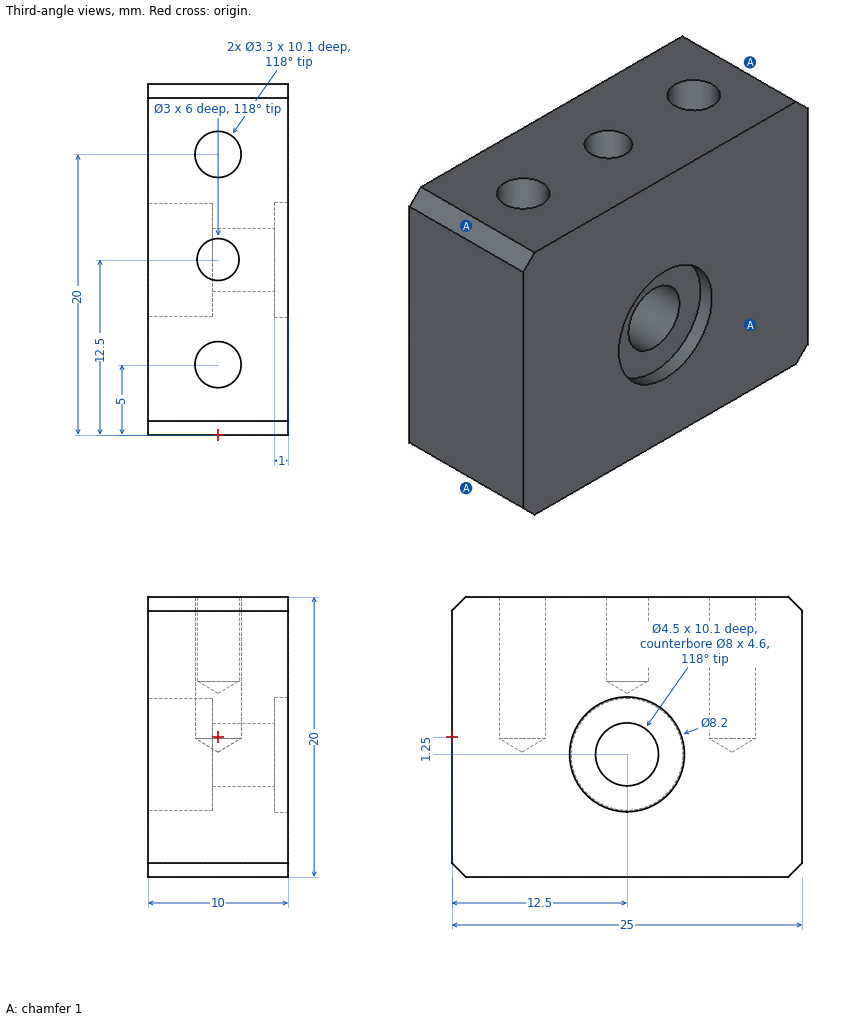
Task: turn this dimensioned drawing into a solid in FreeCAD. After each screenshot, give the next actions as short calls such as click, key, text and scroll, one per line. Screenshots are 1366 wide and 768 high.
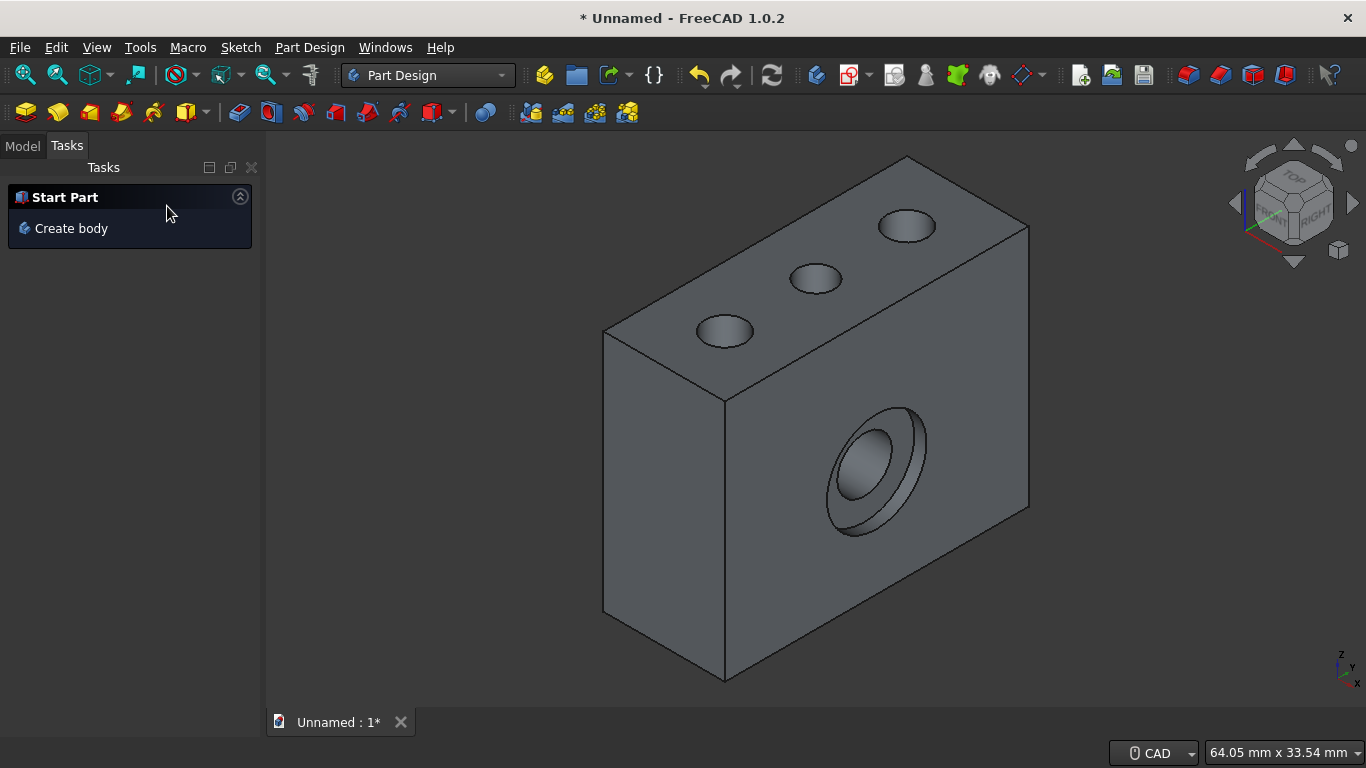
click(664, 365)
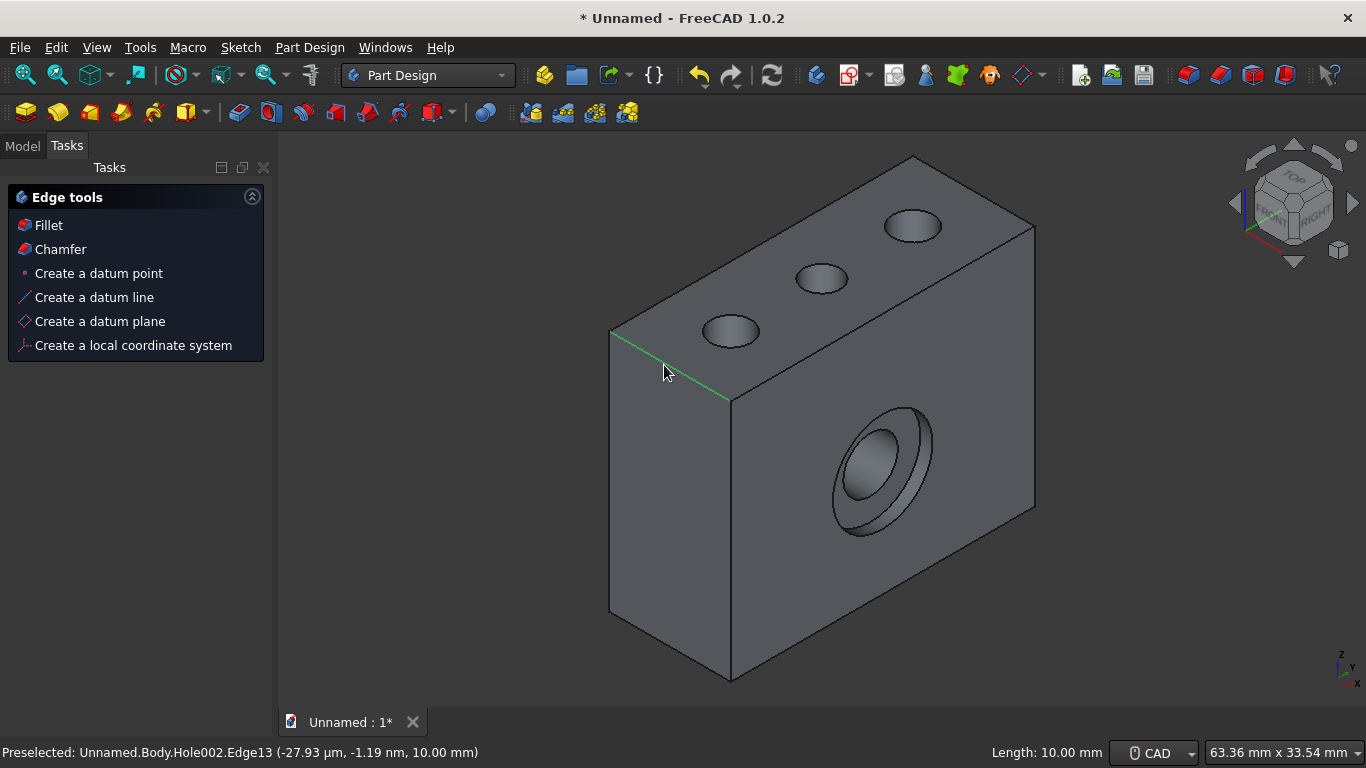
key(2)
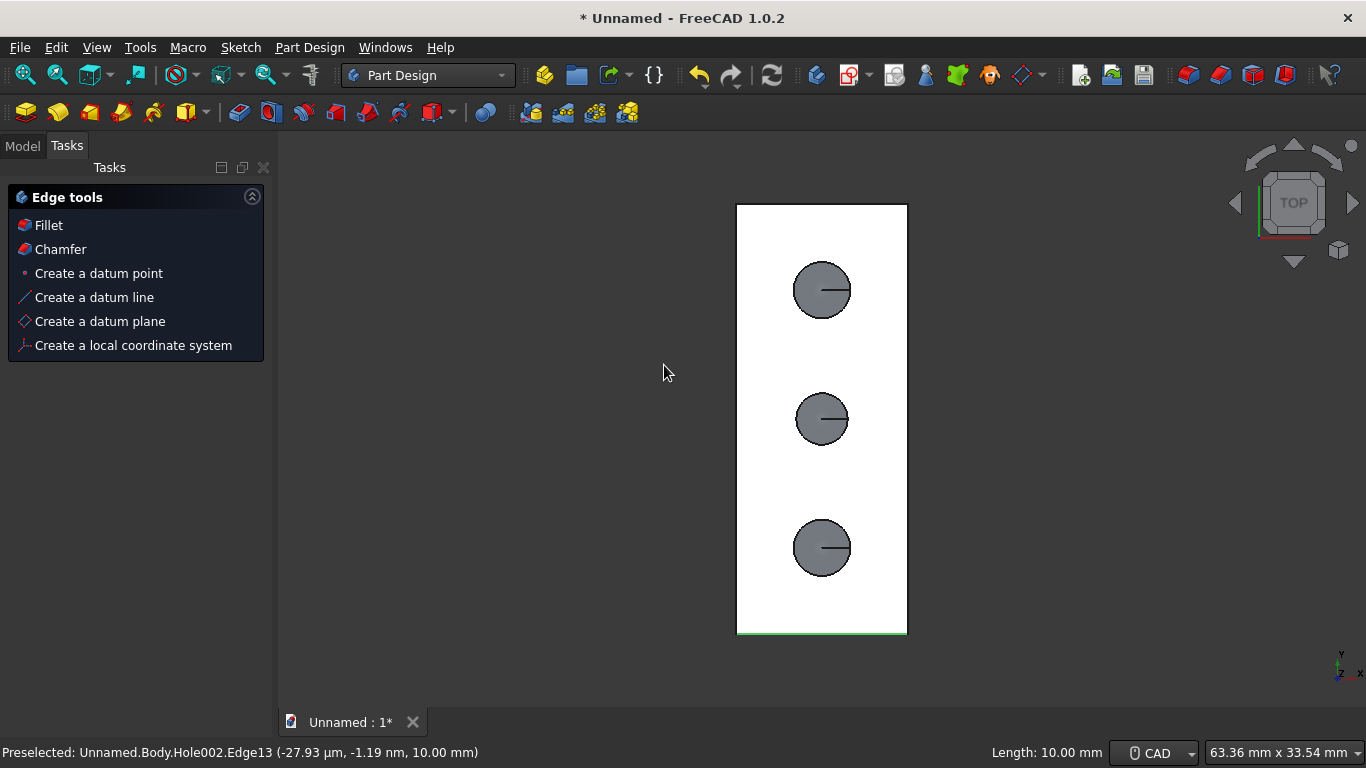
click(822, 203, ctrl)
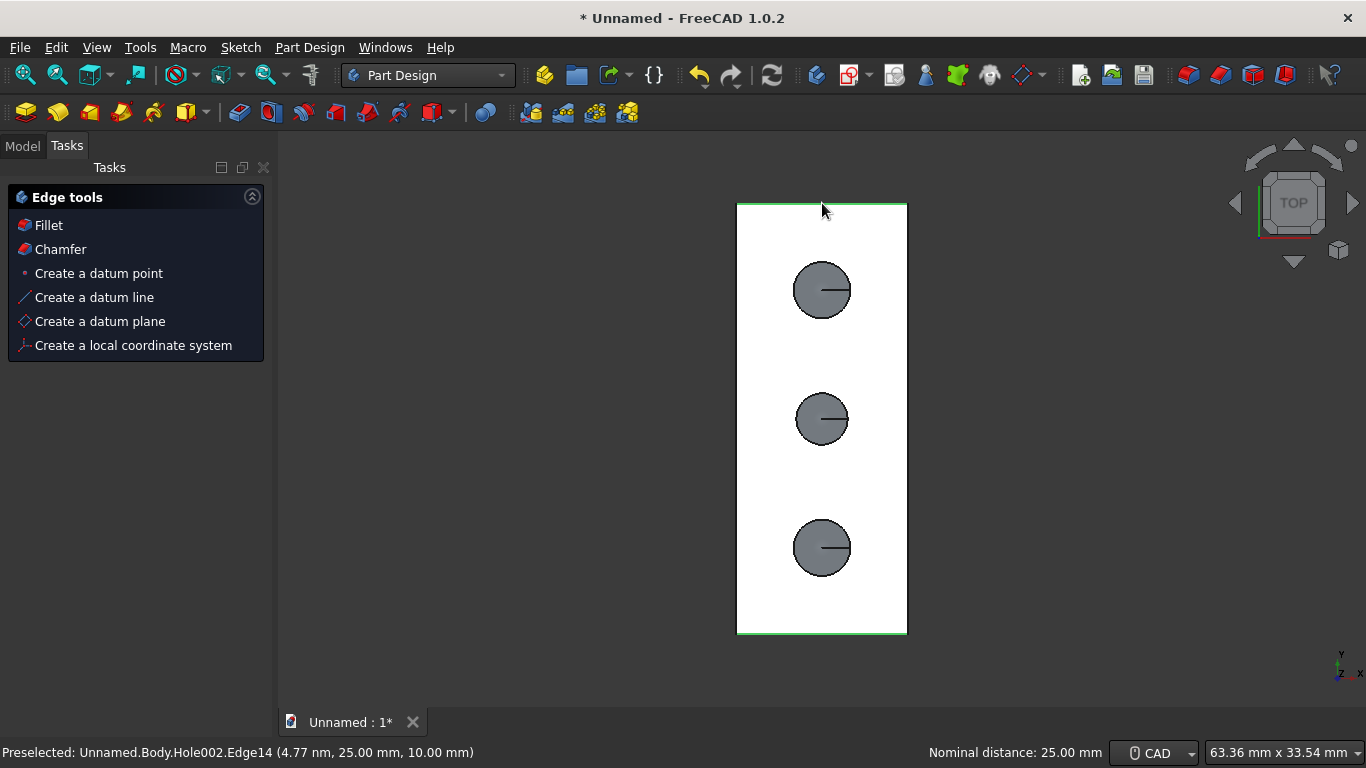
key(0)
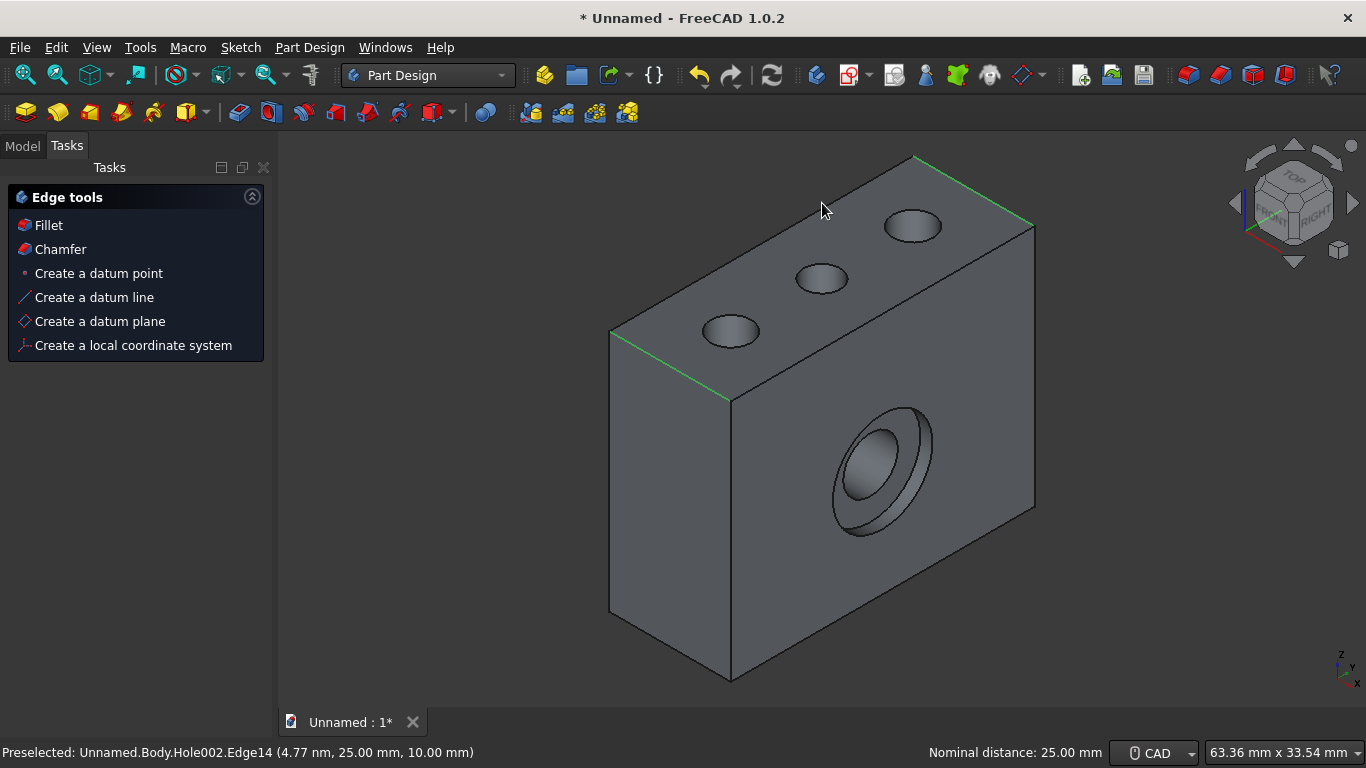
key(1)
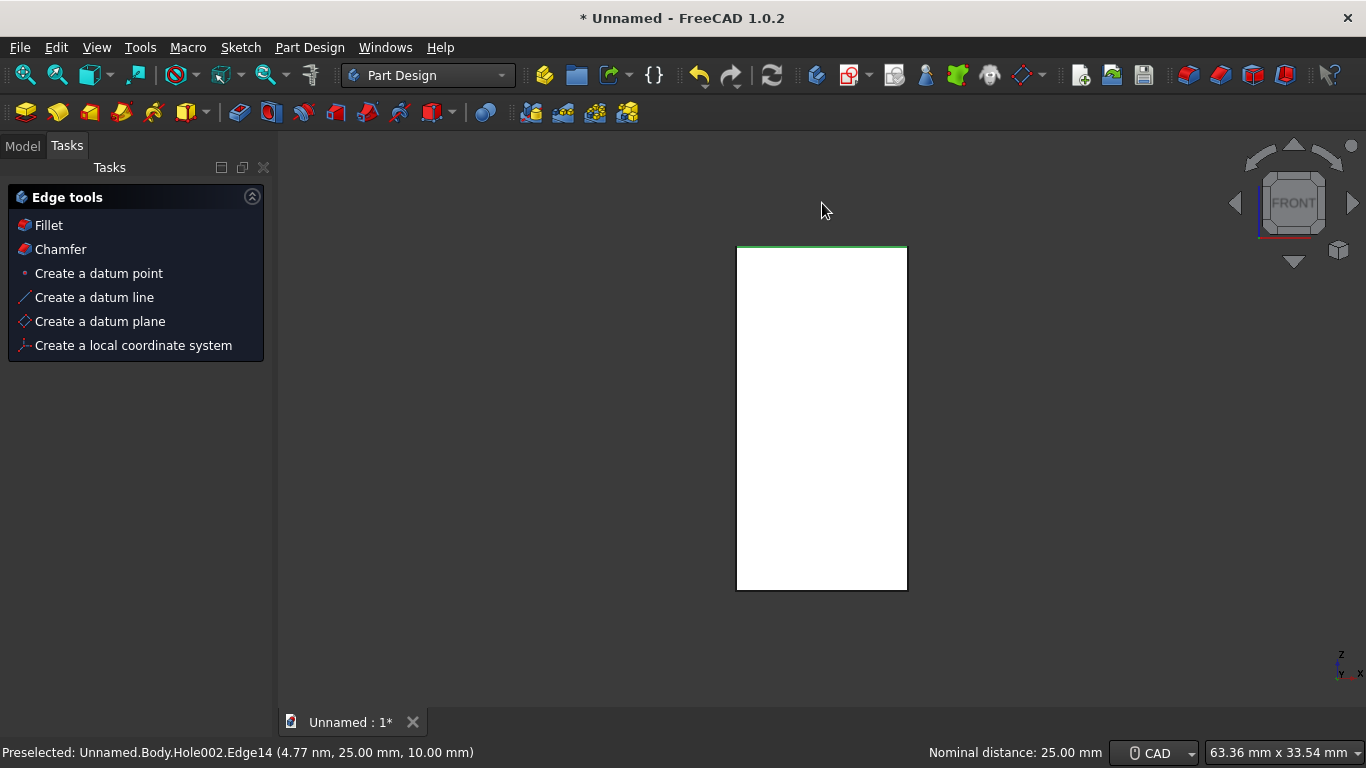
key(3)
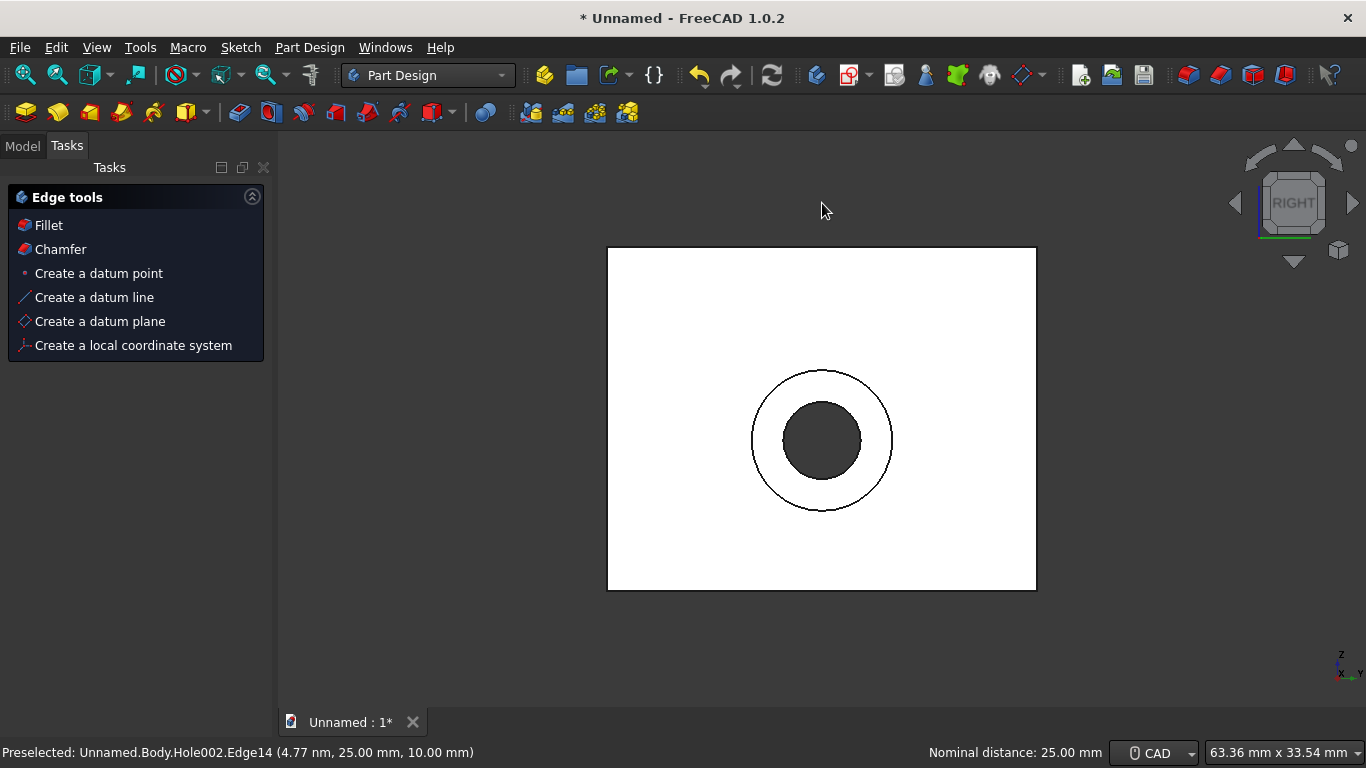
key(5)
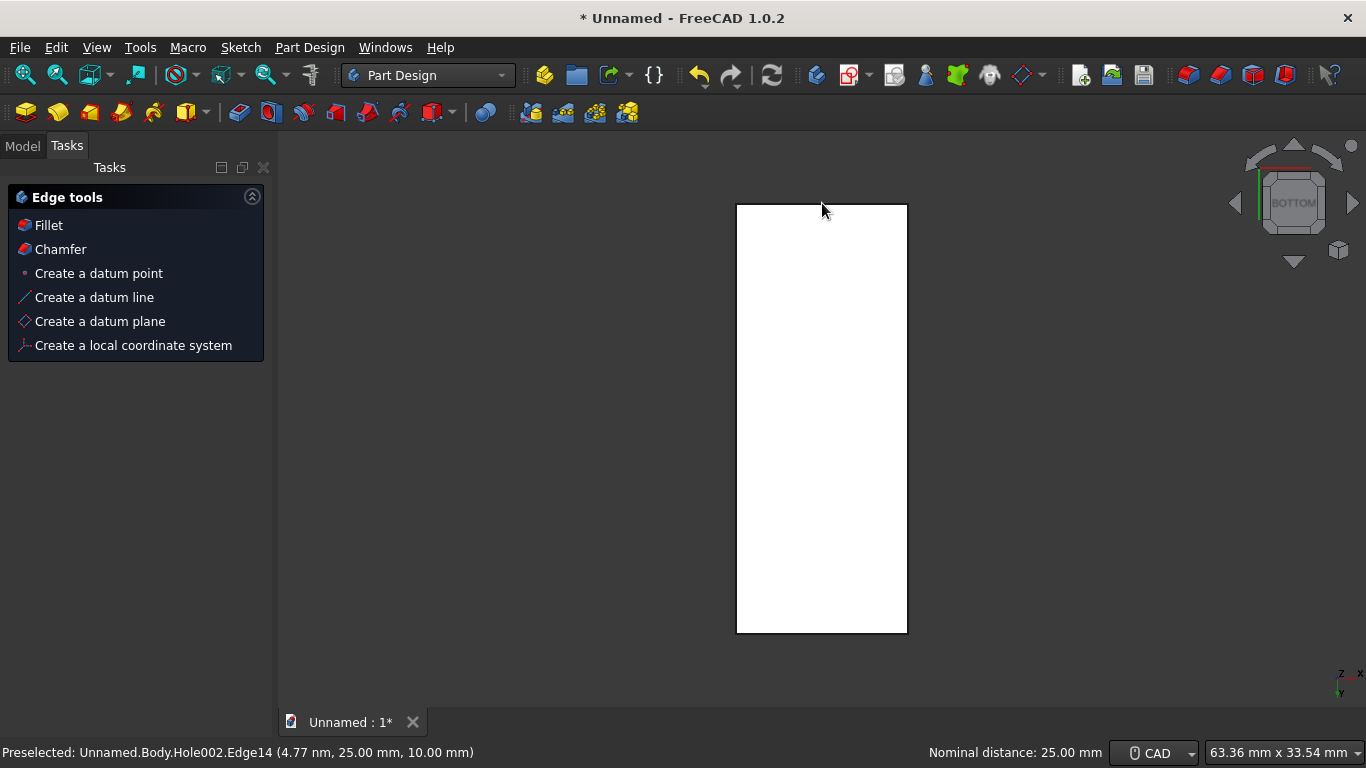
click(822, 203, ctrl)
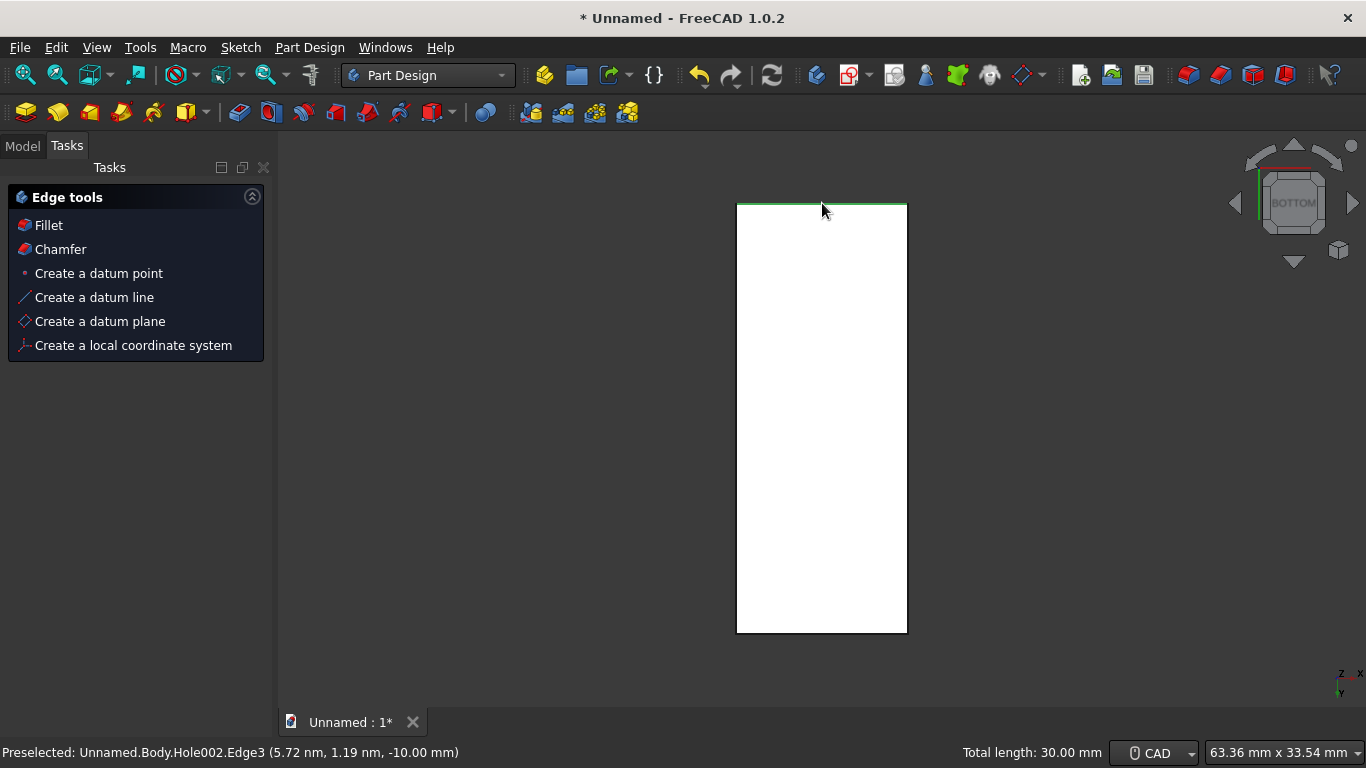
key(4)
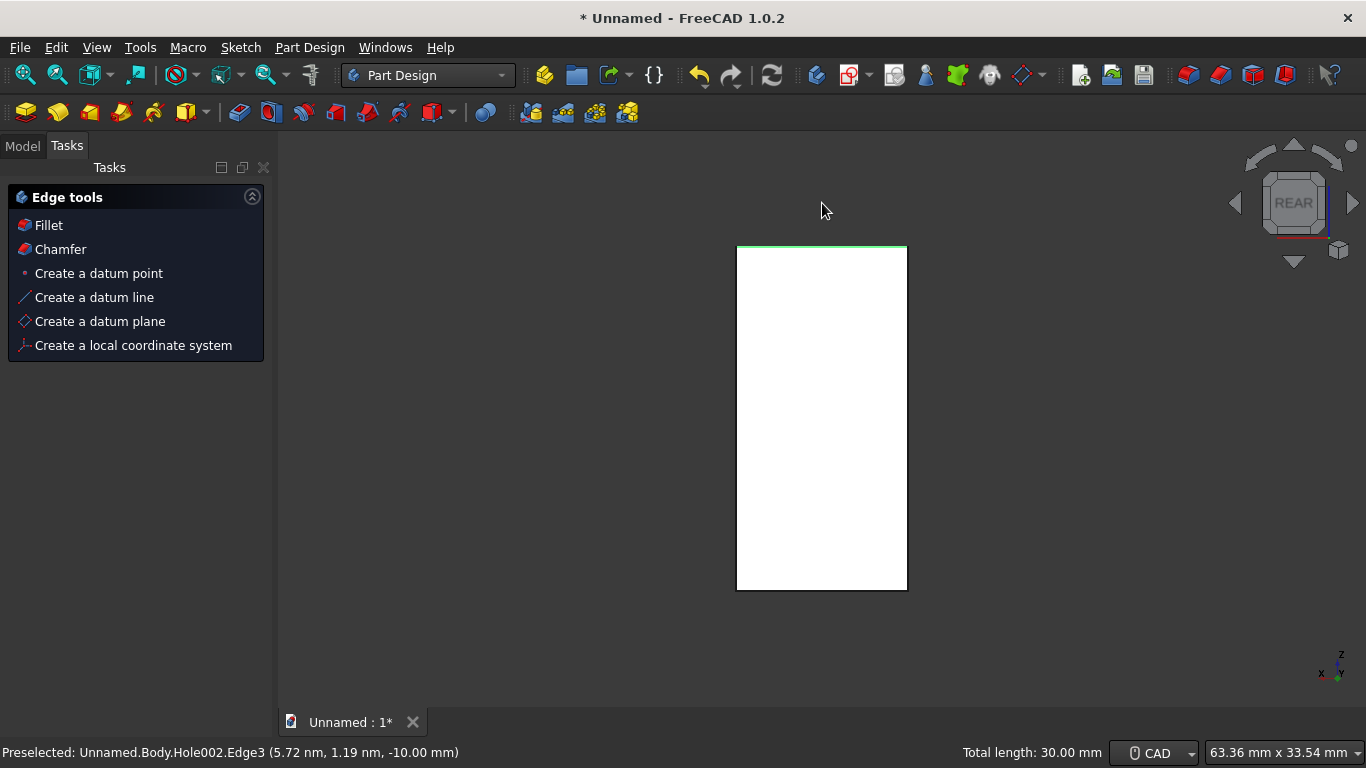
click(822, 590, ctrl)